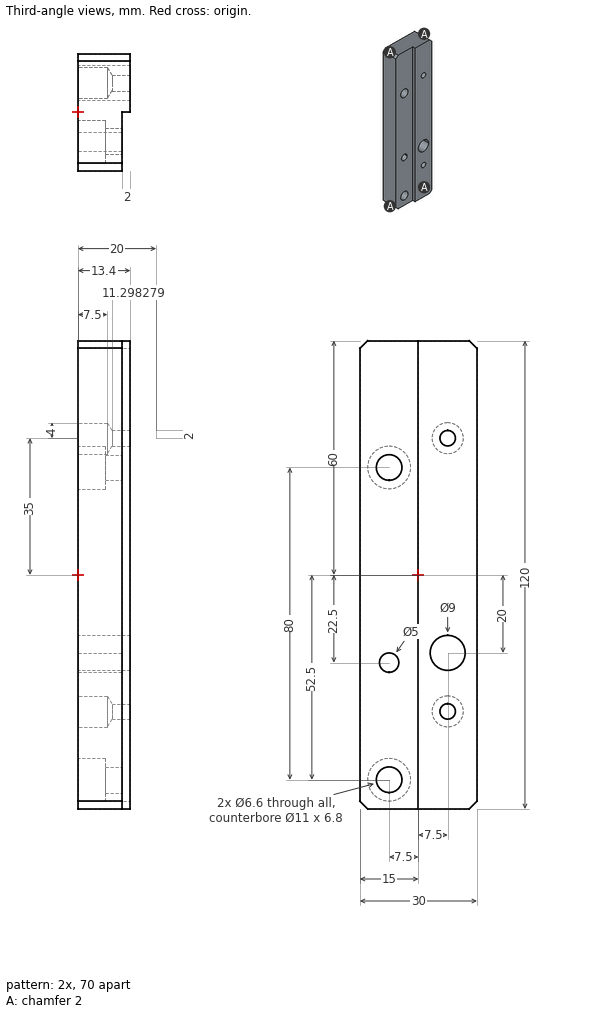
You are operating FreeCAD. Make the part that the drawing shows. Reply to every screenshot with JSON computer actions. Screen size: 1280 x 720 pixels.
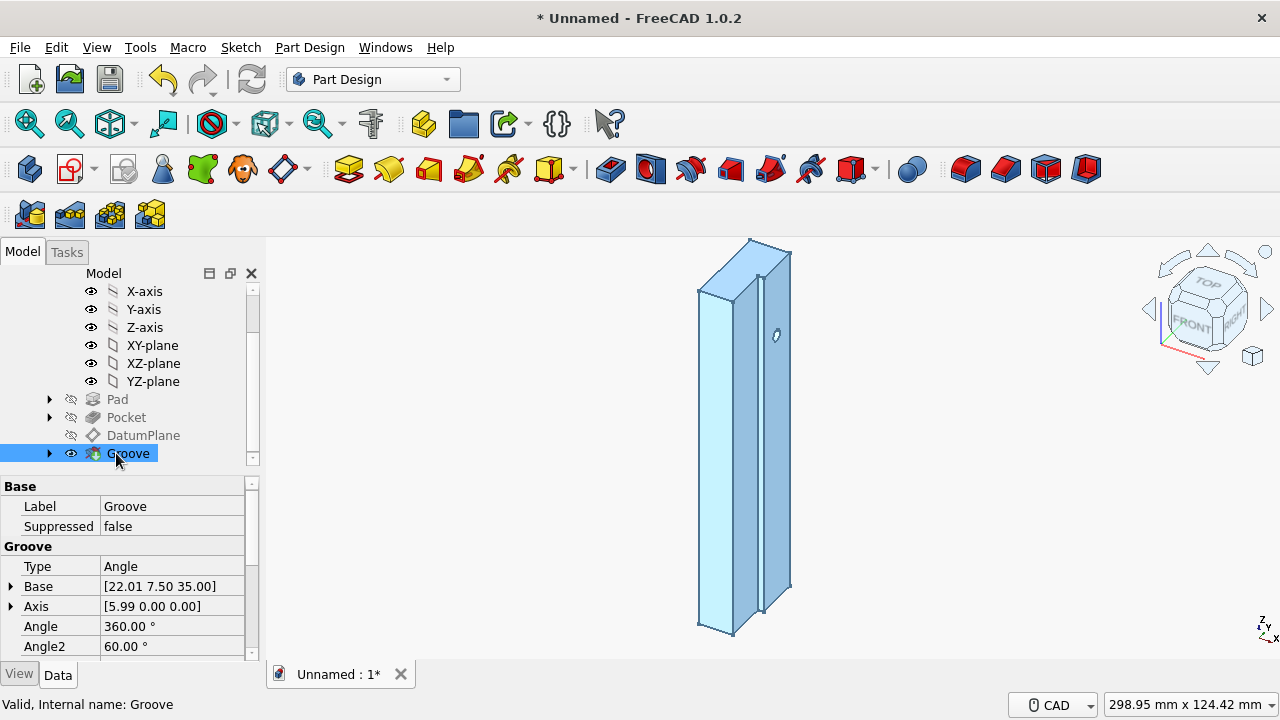
{"action": "left_click", "coordinate": [70, 214]}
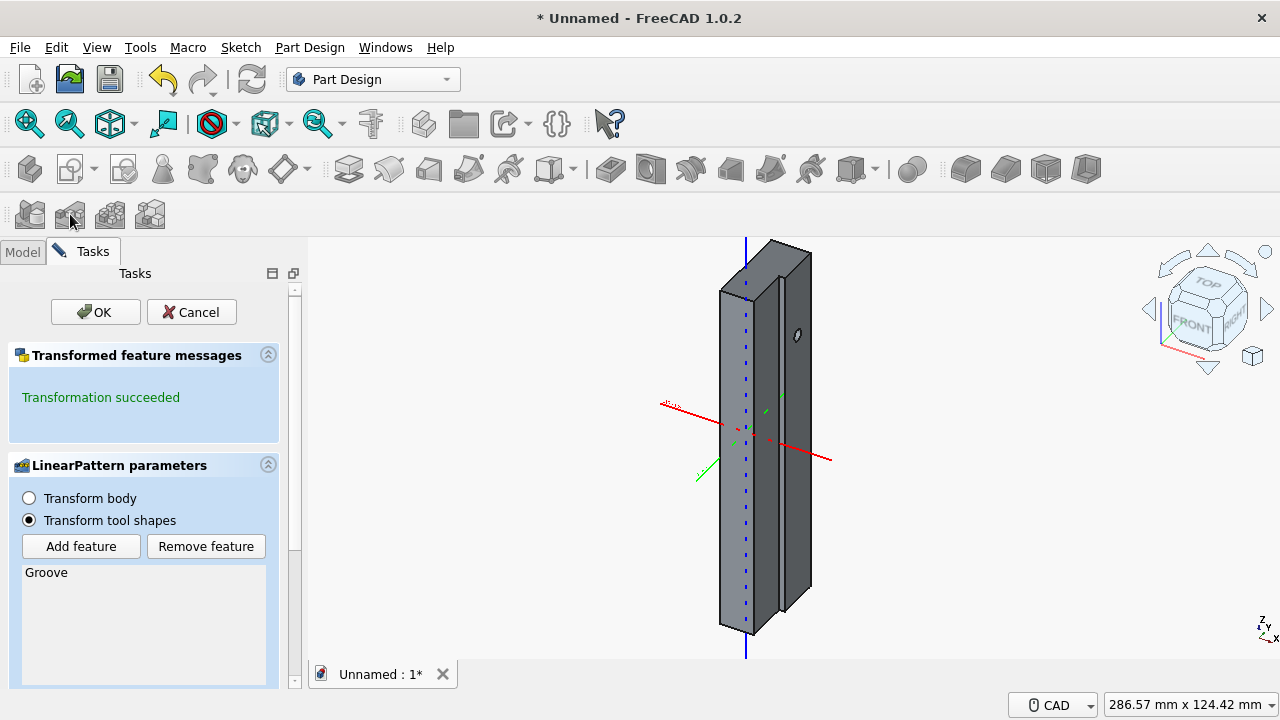
{"action": "scroll", "coordinate": [295, 486], "scroll_direction": "down", "scroll_amount": 2}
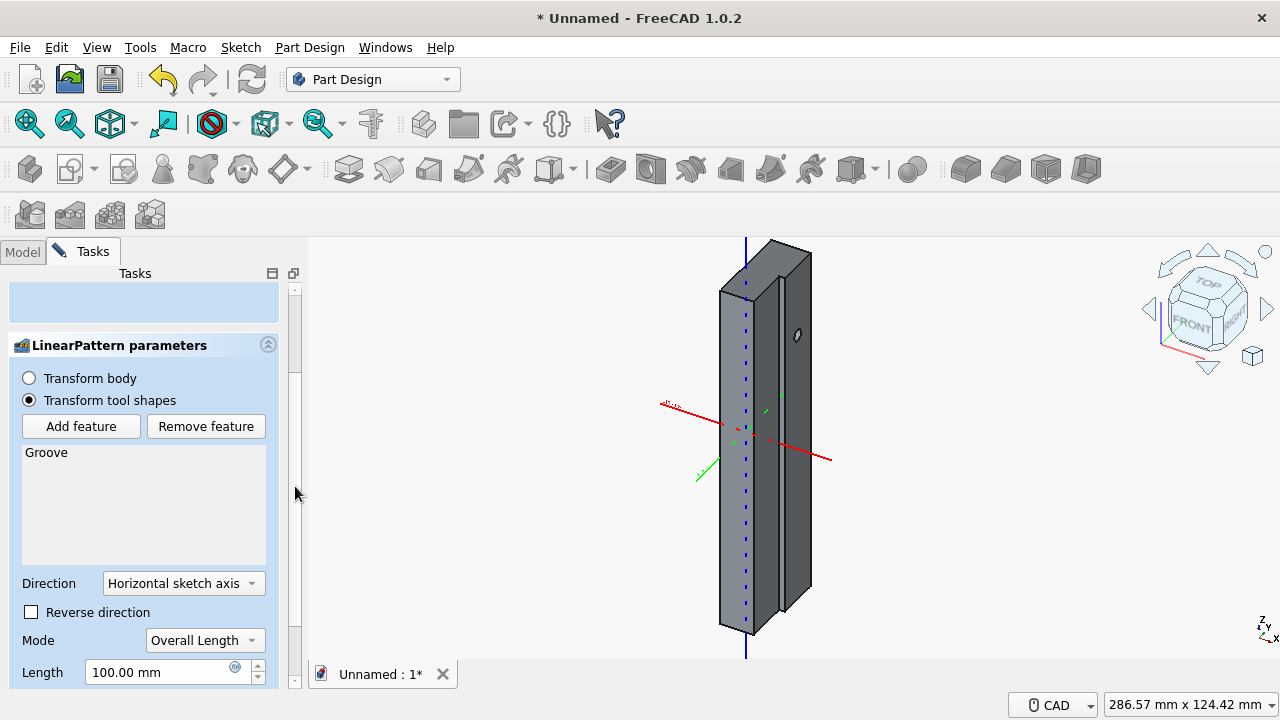
{"action": "left_click", "coordinate": [184, 584]}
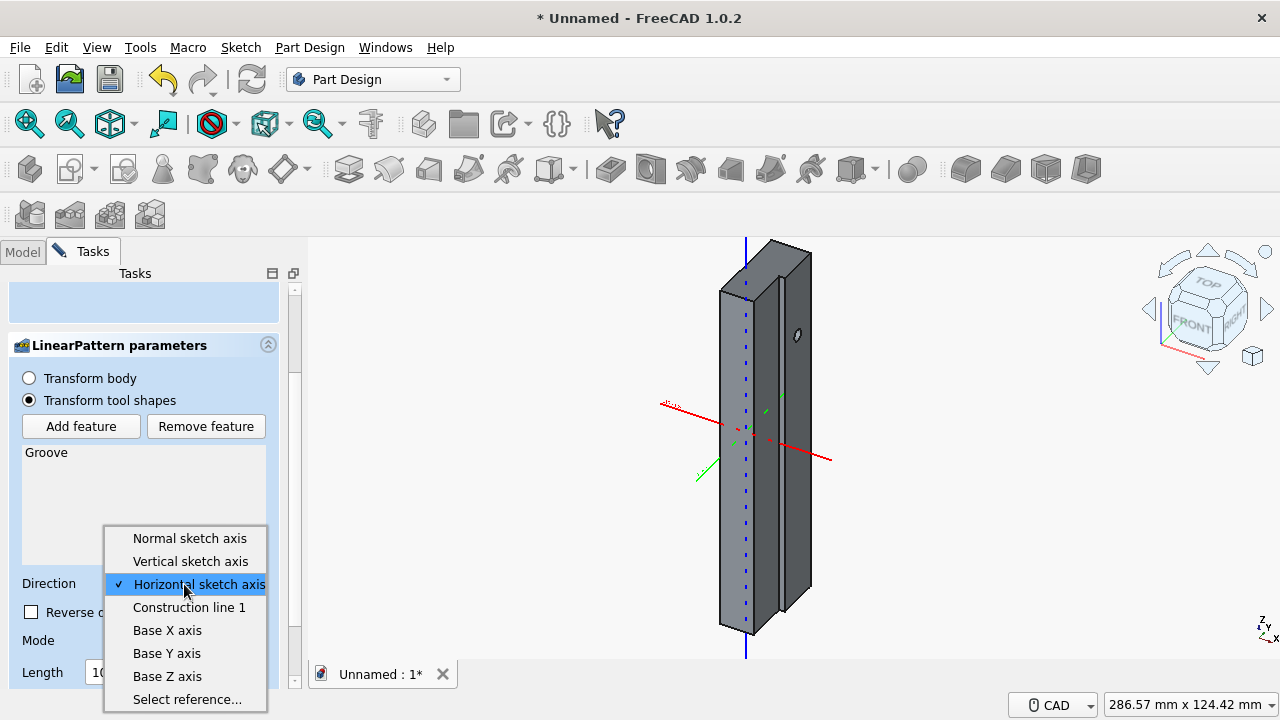
{"action": "left_click", "coordinate": [184, 676]}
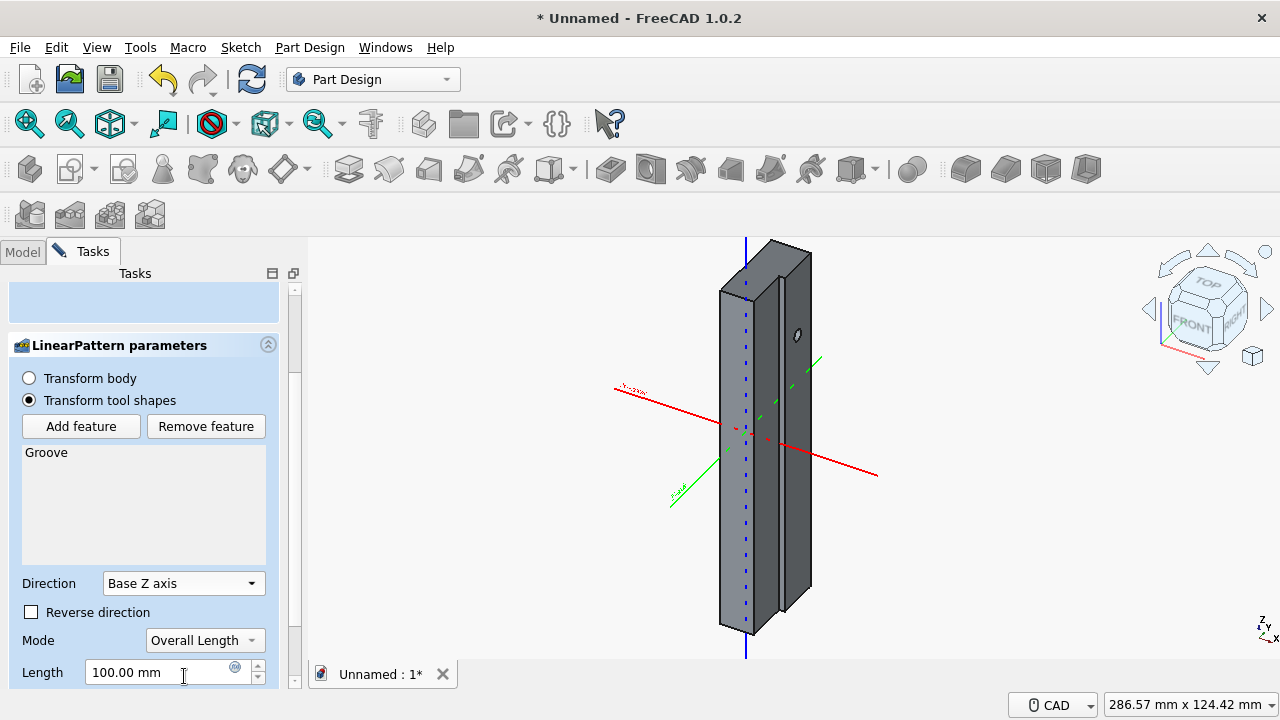
{"action": "left_click", "coordinate": [206, 640]}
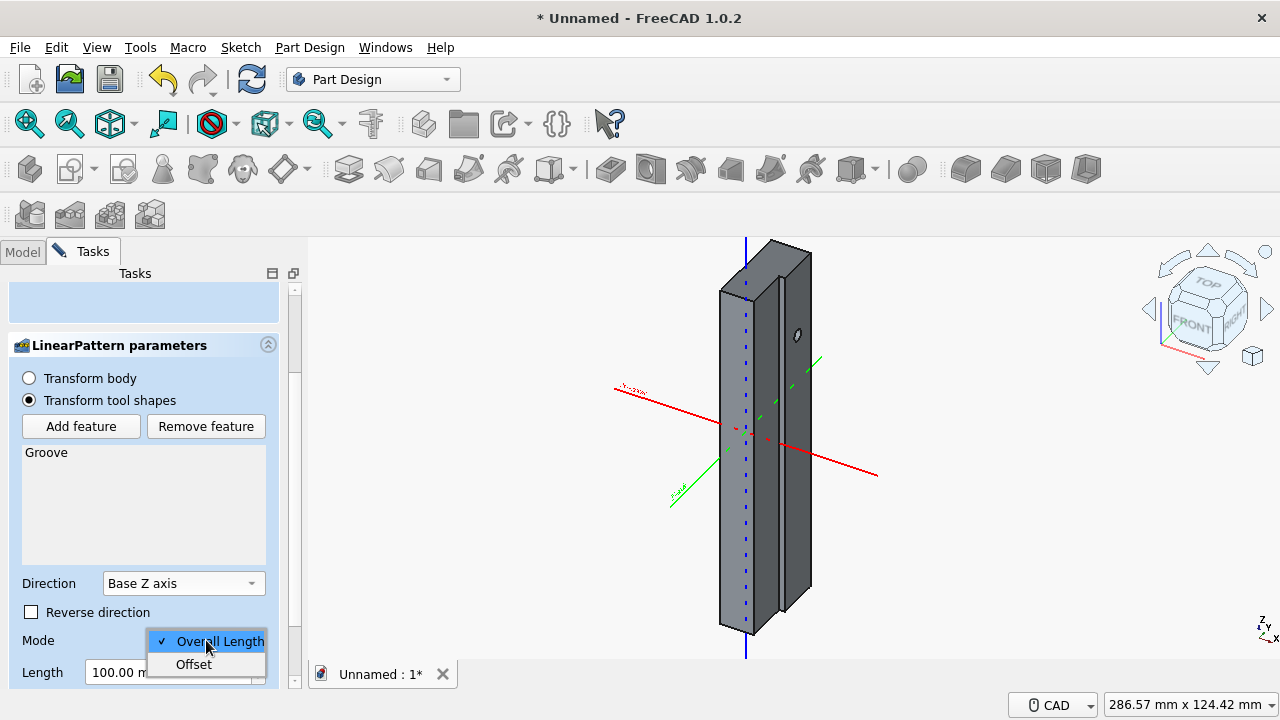
{"action": "left_click", "coordinate": [206, 664]}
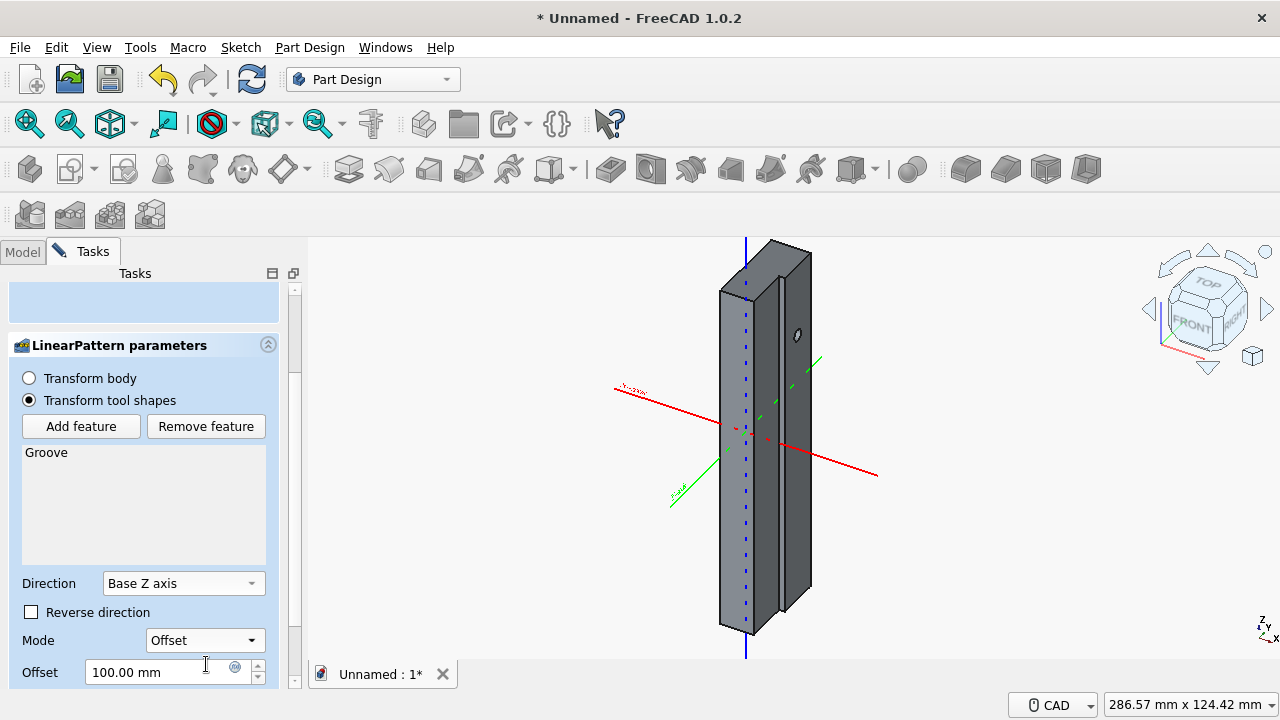
{"action": "triple_click", "coordinate": [168, 672]}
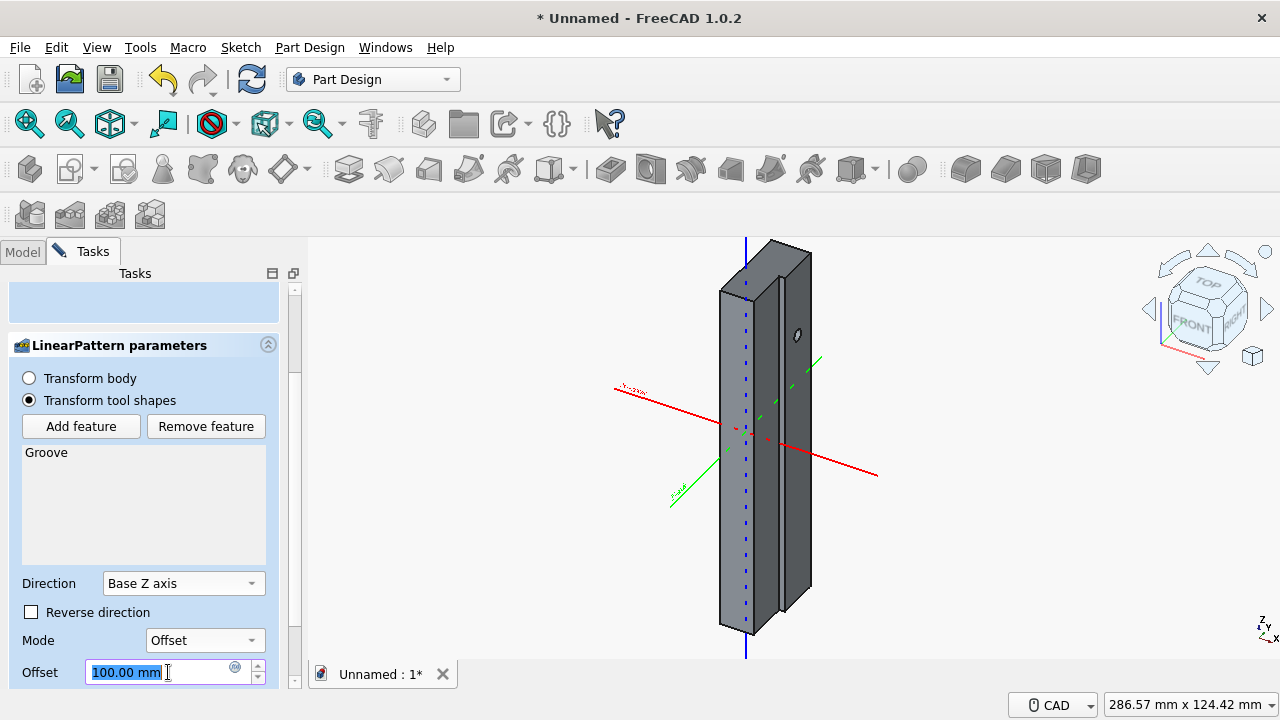
{"action": "type", "text": "70"}
{"action": "key", "text": "Tab"}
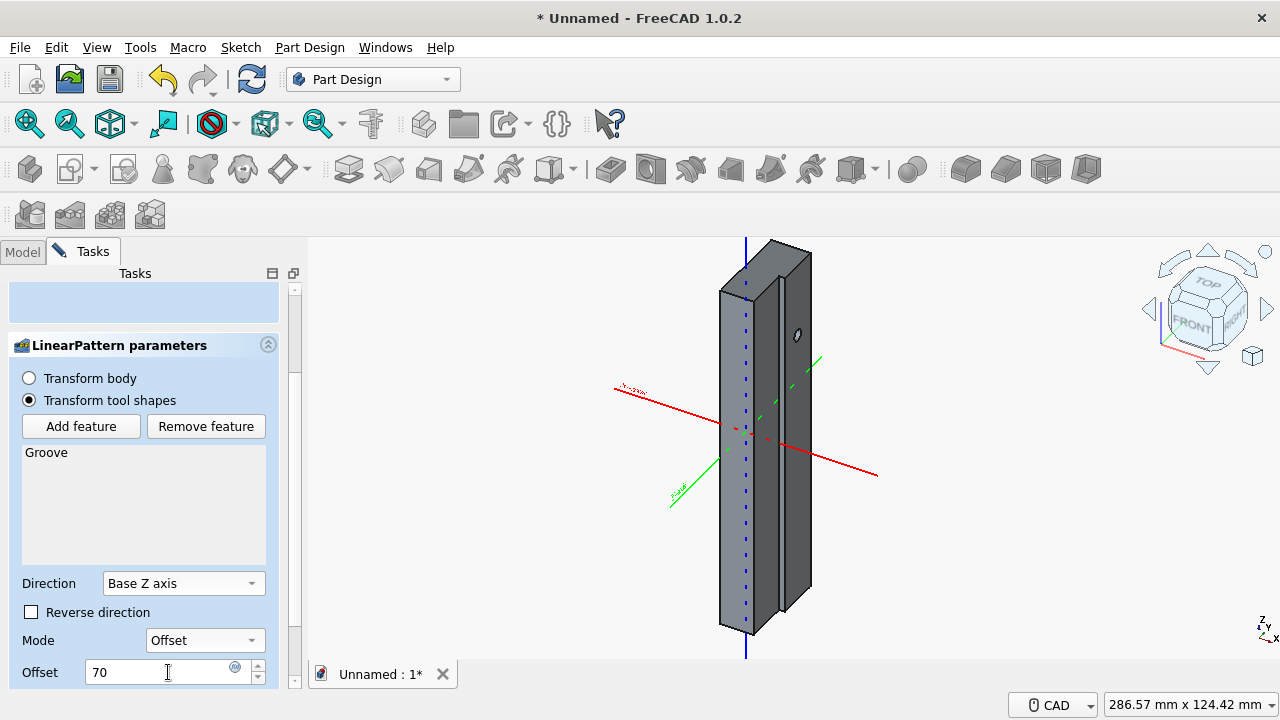
{"action": "scroll", "coordinate": [295, 486], "scroll_direction": "down", "scroll_amount": 2}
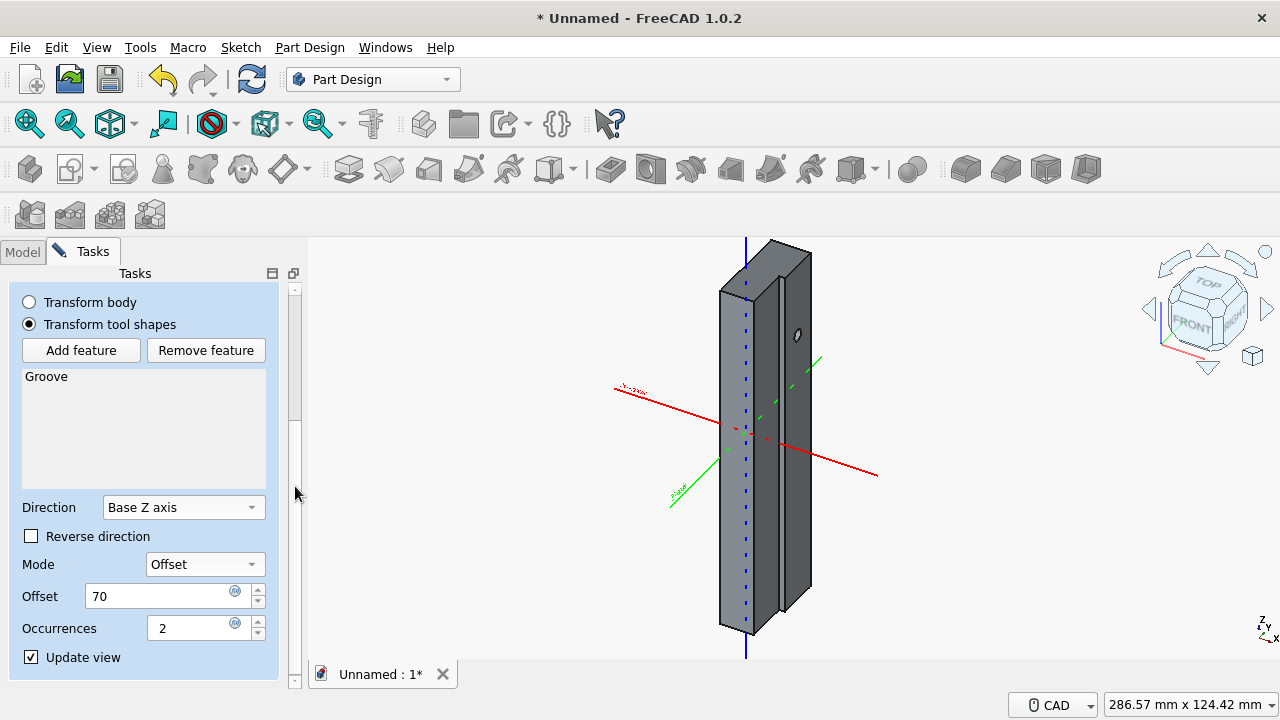
{"action": "triple_click", "coordinate": [198, 628]}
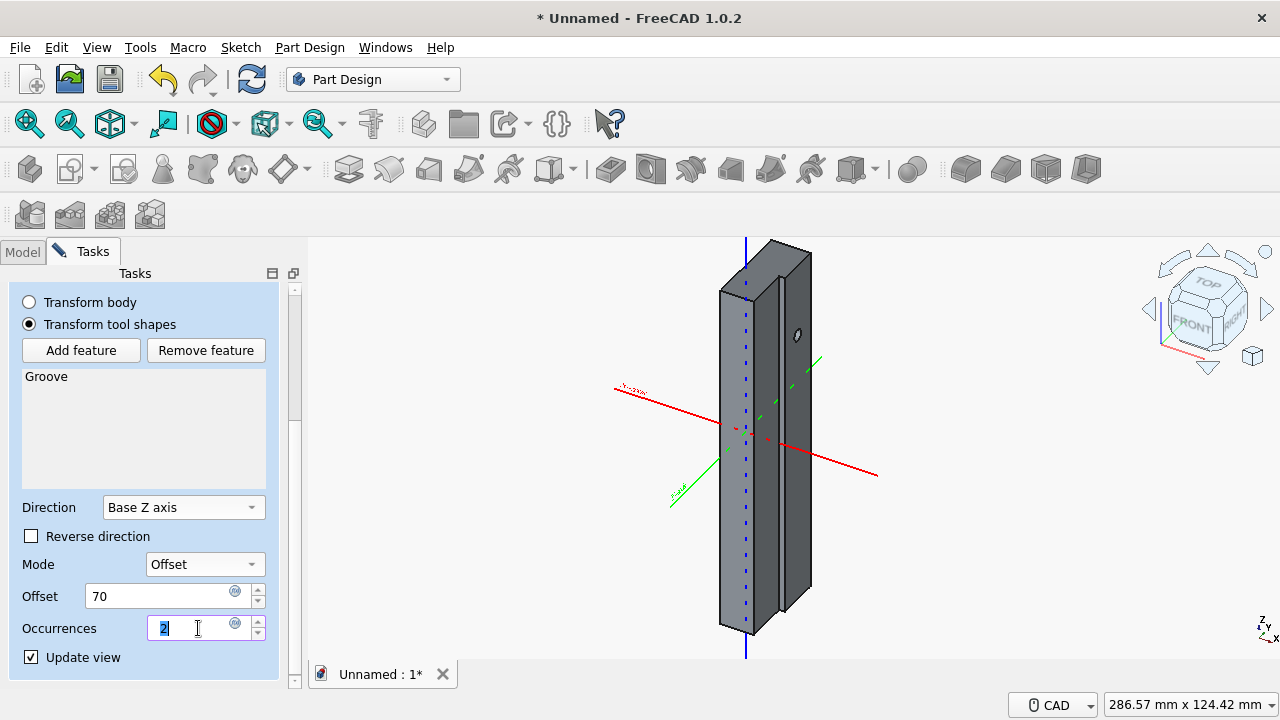
{"action": "type", "text": "2"}
{"action": "key", "text": "Tab"}